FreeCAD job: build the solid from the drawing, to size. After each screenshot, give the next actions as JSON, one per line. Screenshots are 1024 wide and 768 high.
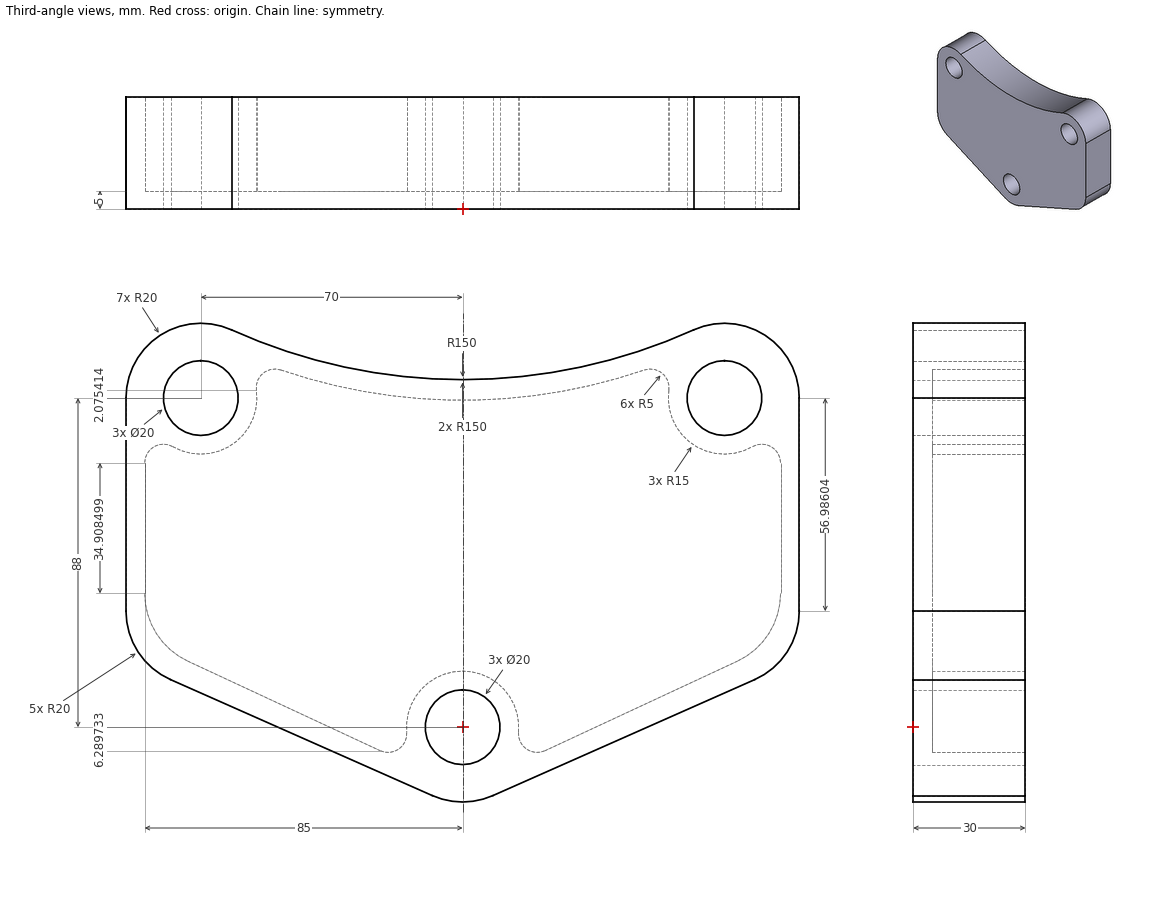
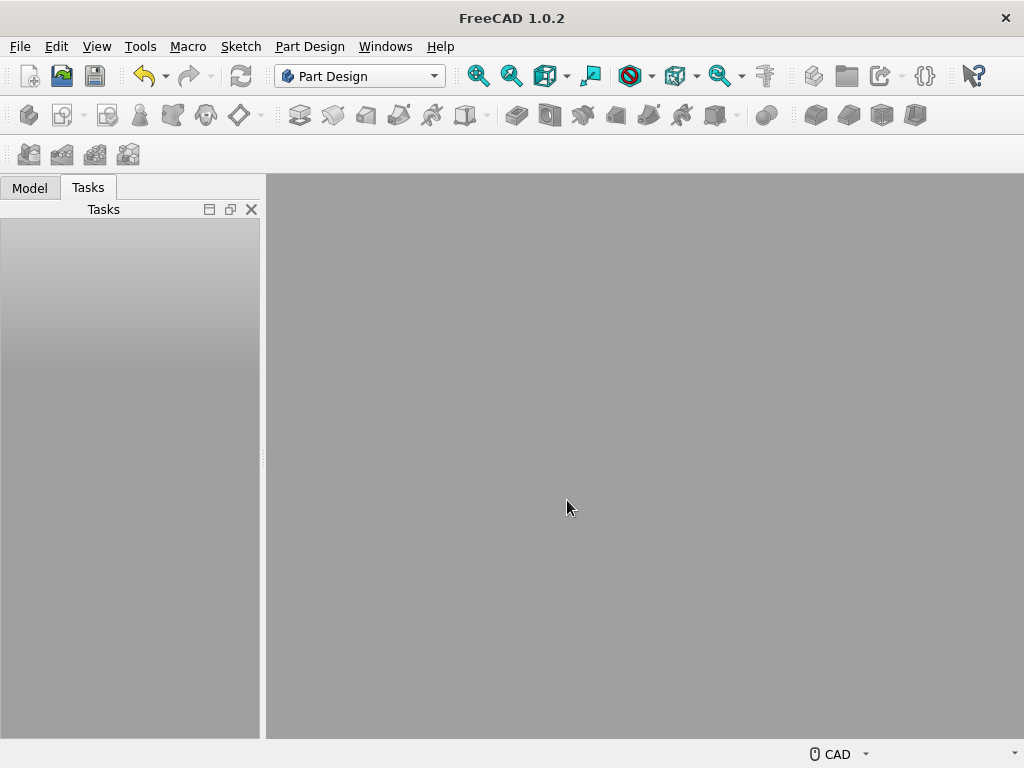
{"action": "left_click", "coordinate": [29, 76]}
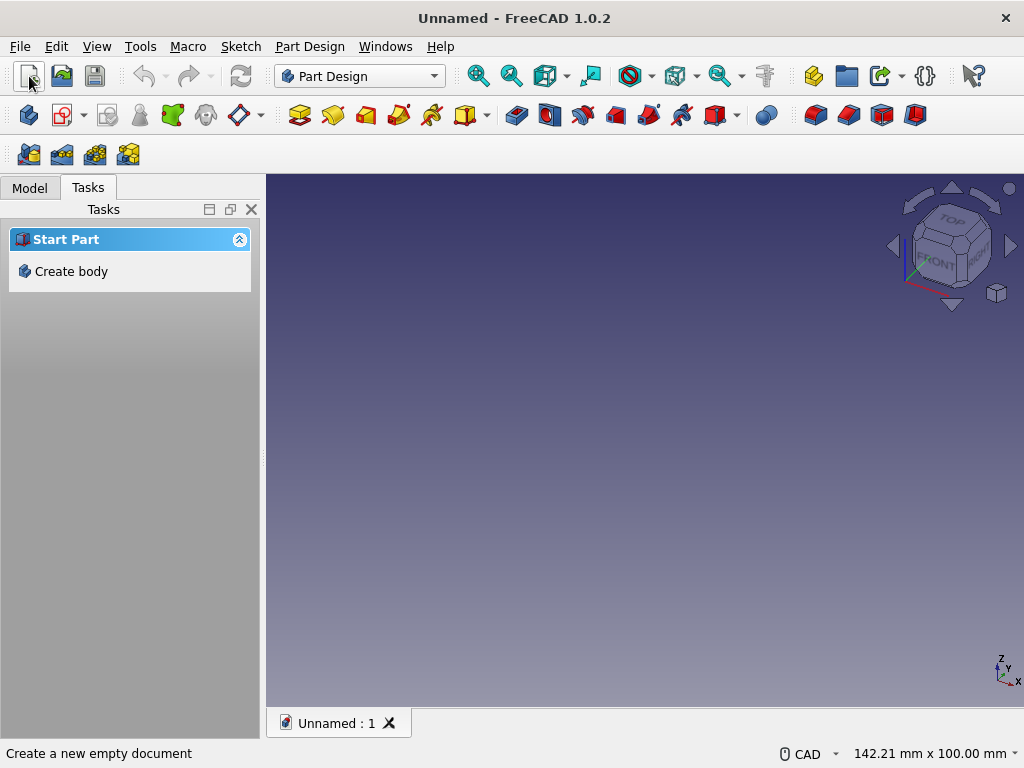
{"action": "left_click", "coordinate": [62, 116]}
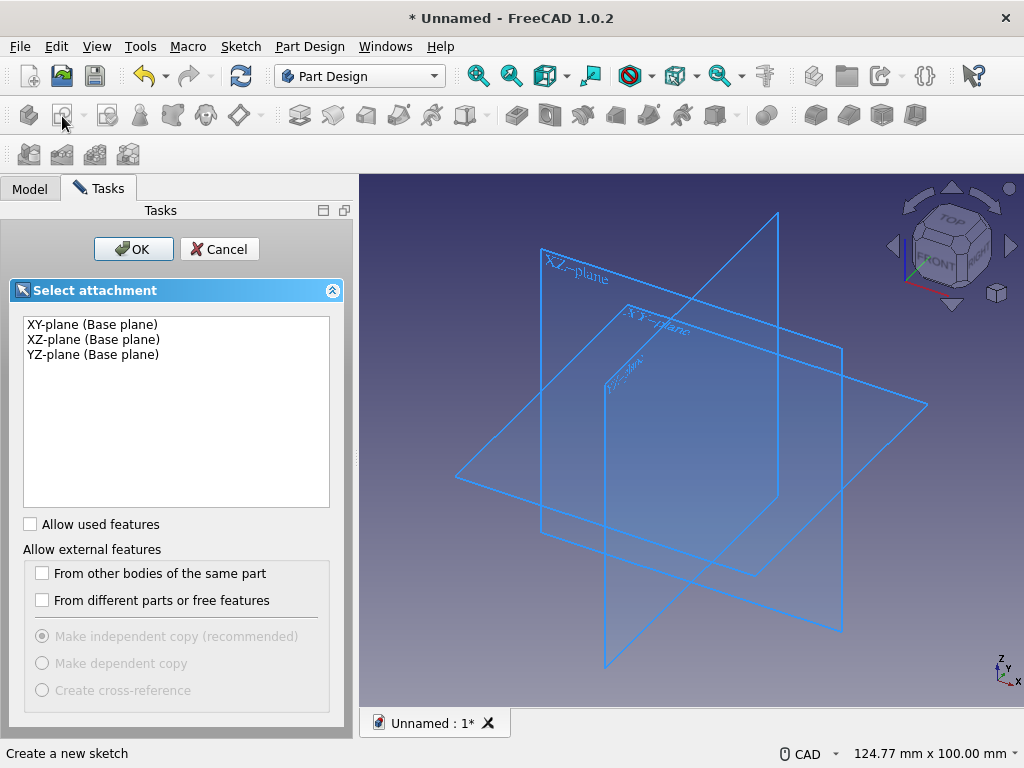
{"action": "left_click", "coordinate": [84, 340]}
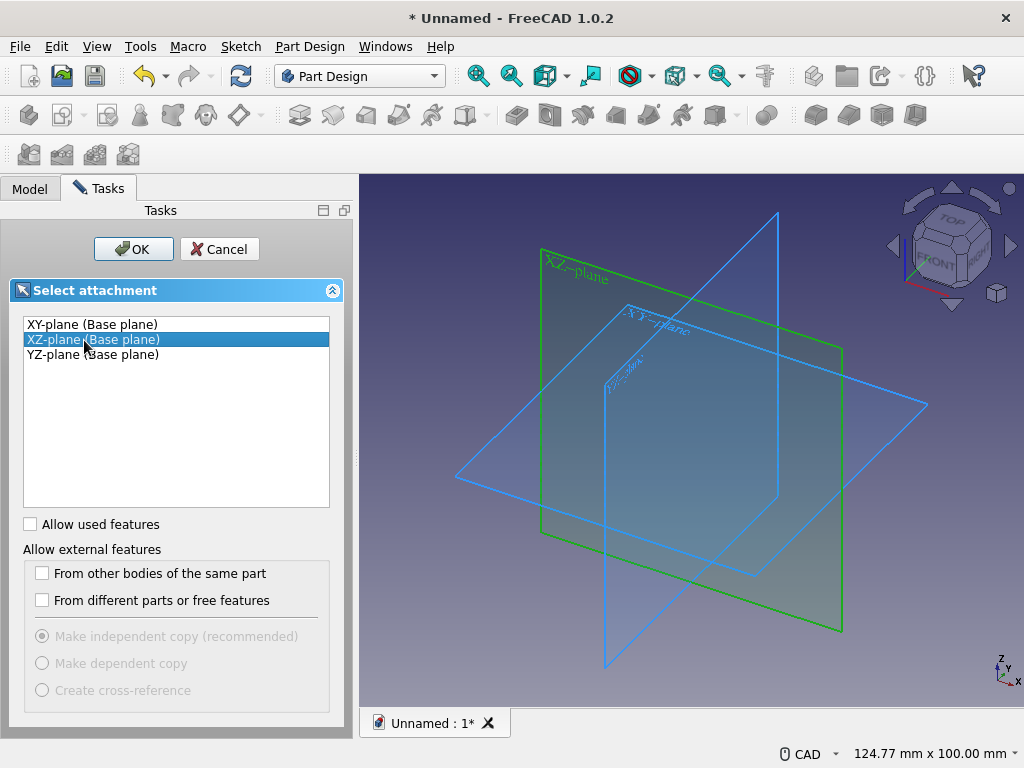
{"action": "left_click", "coordinate": [134, 249]}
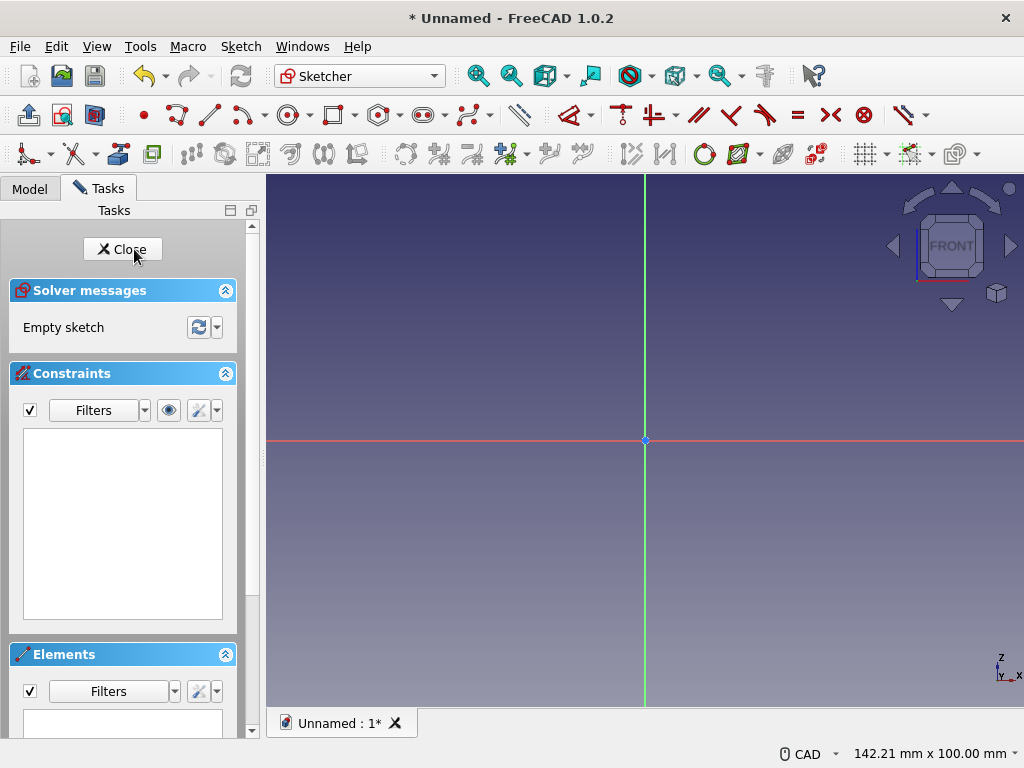
{"action": "scroll", "coordinate": [521, 628], "scroll_direction": "down", "scroll_amount": 4}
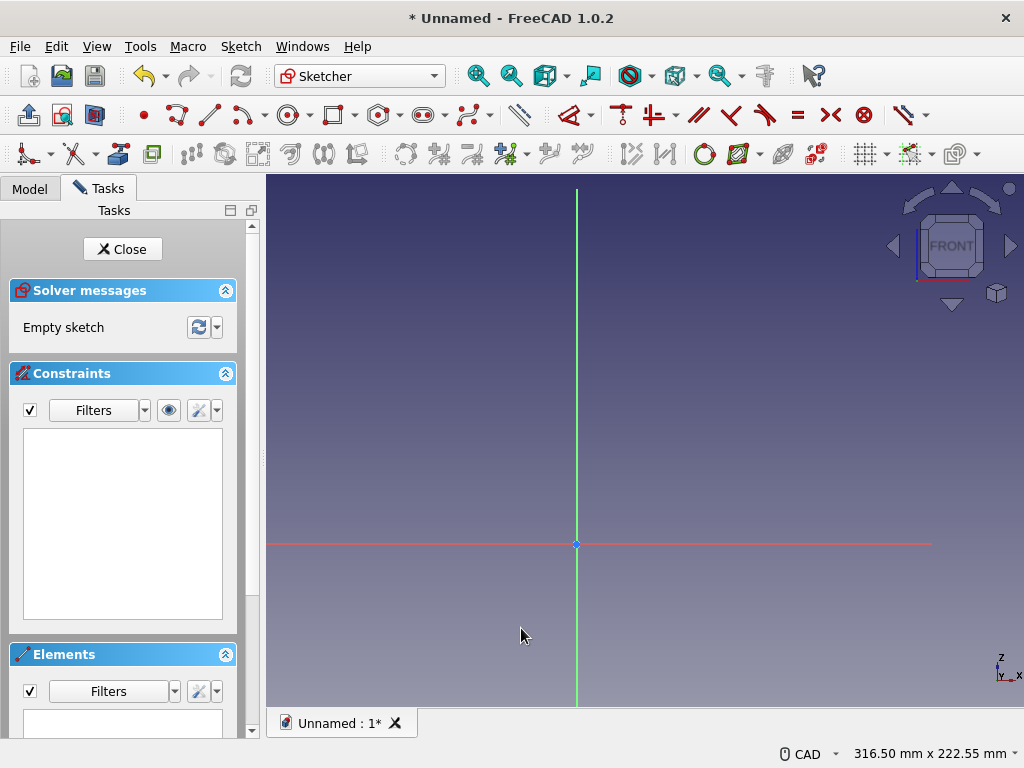
{"action": "left_click", "coordinate": [210, 116]}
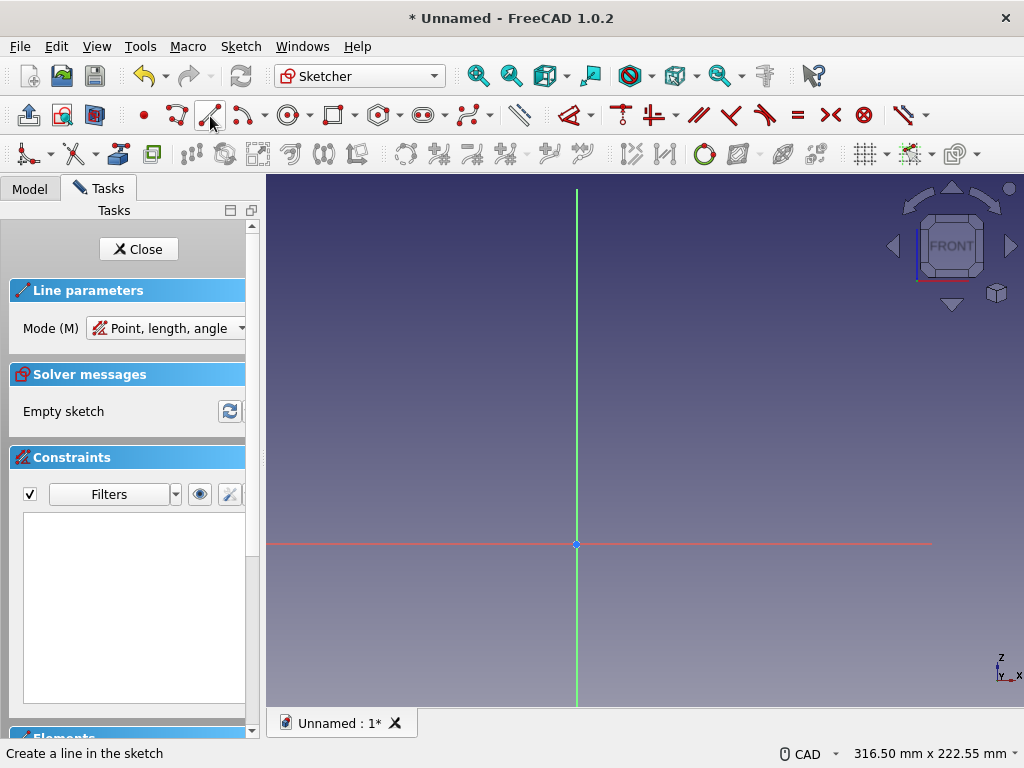
{"action": "left_click", "coordinate": [792, 333]}
{"action": "left_click", "coordinate": [792, 470]}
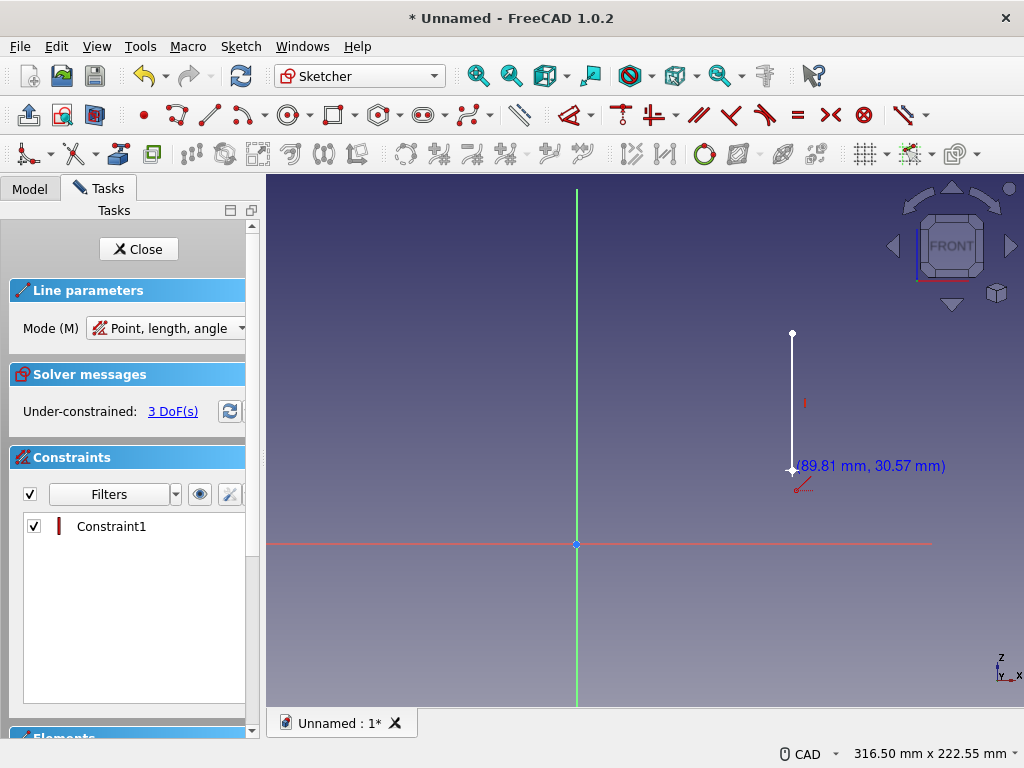
{"action": "left_click", "coordinate": [764, 514]}
{"action": "left_click", "coordinate": [596, 588]}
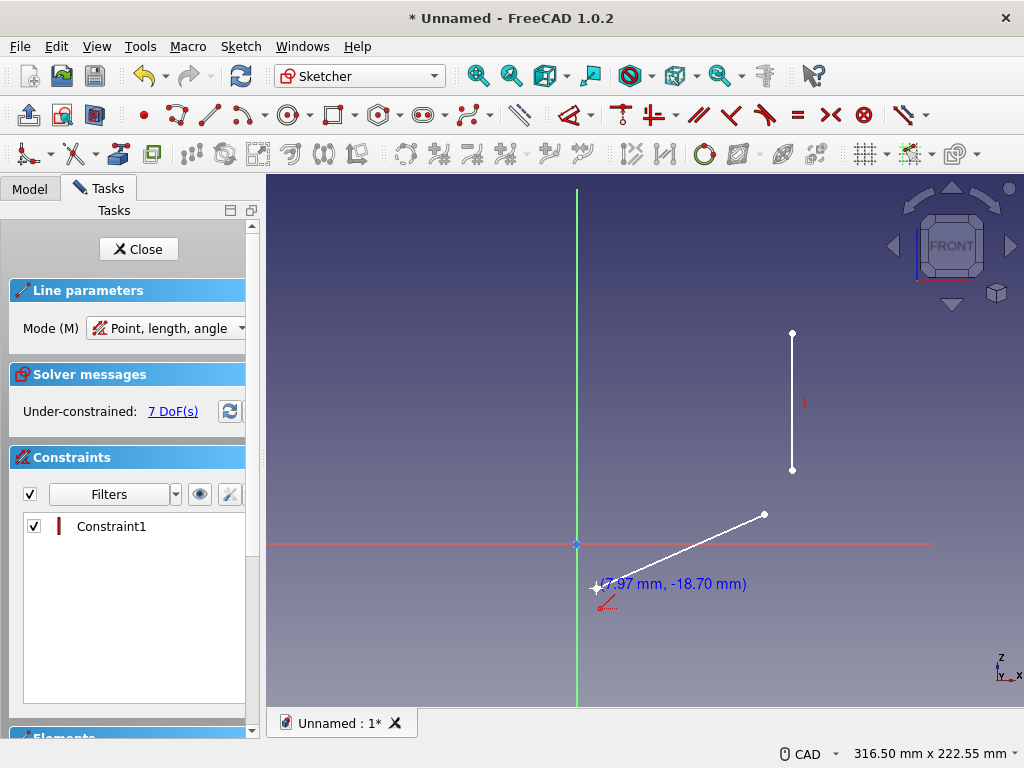
{"action": "left_click", "coordinate": [557, 588]}
{"action": "left_click", "coordinate": [390, 514]}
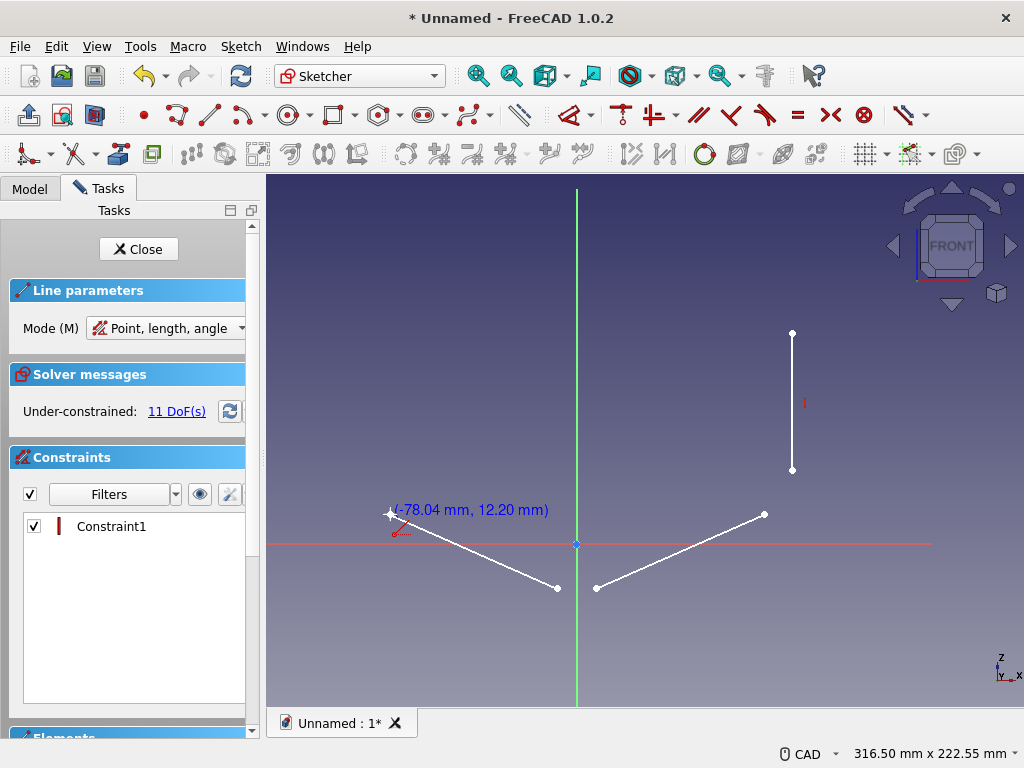
{"action": "left_click", "coordinate": [361, 470]}
{"action": "left_click", "coordinate": [361, 333]}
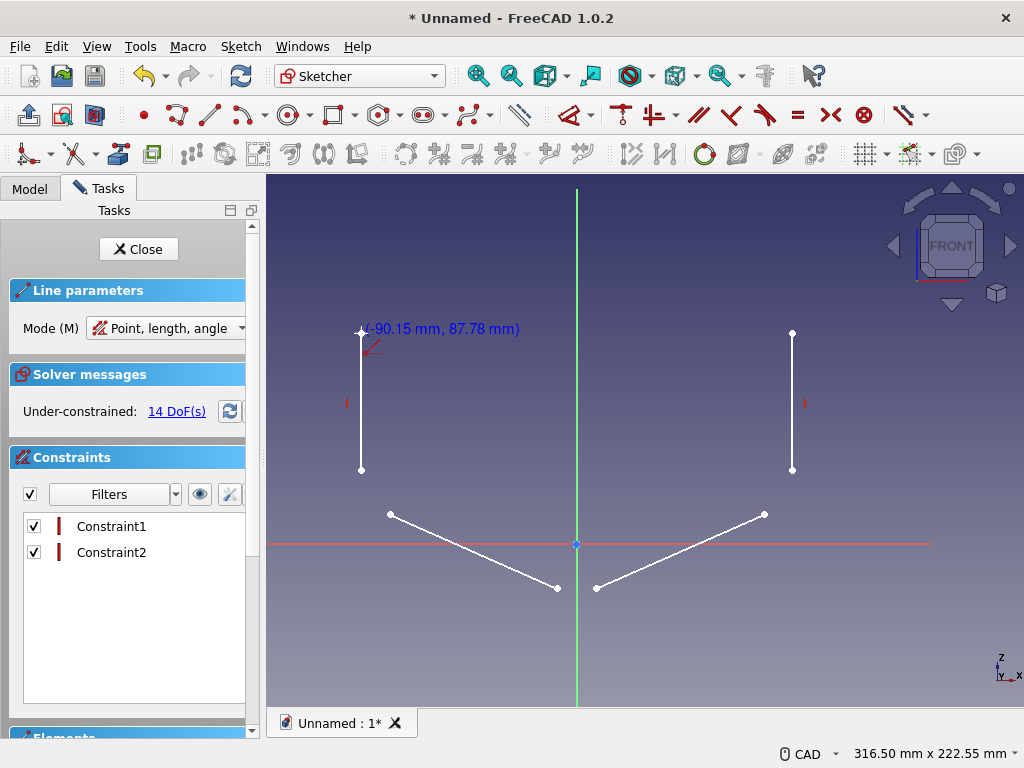
{"action": "left_click", "coordinate": [264, 116]}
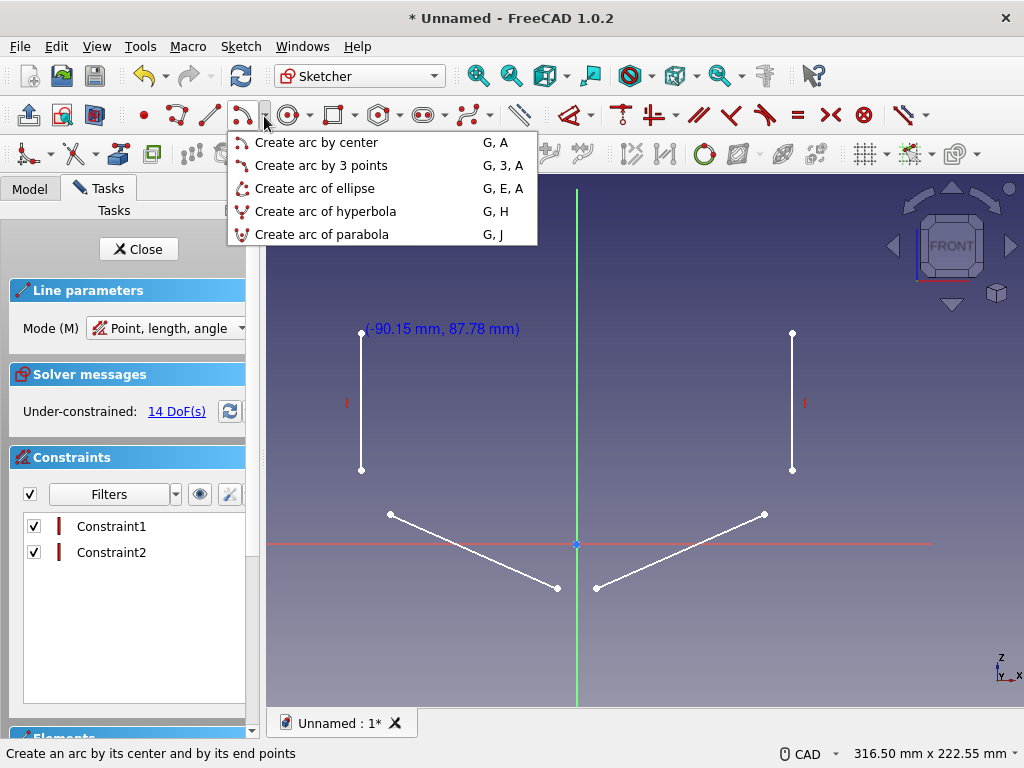
{"action": "left_click", "coordinate": [382, 166]}